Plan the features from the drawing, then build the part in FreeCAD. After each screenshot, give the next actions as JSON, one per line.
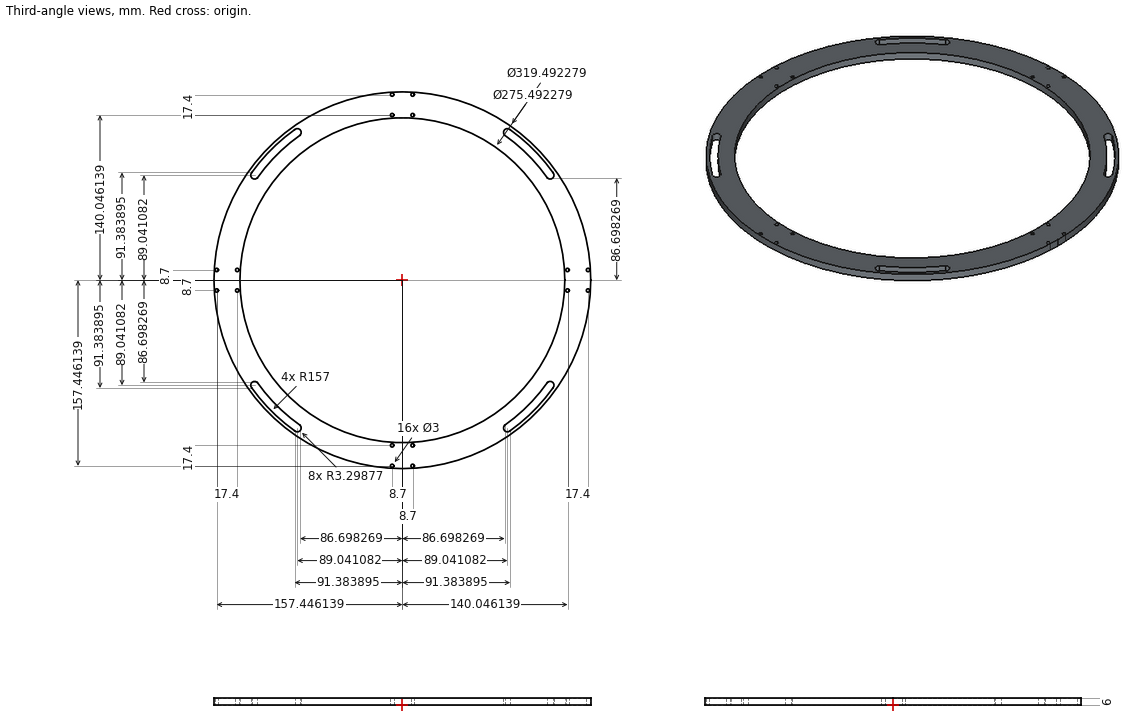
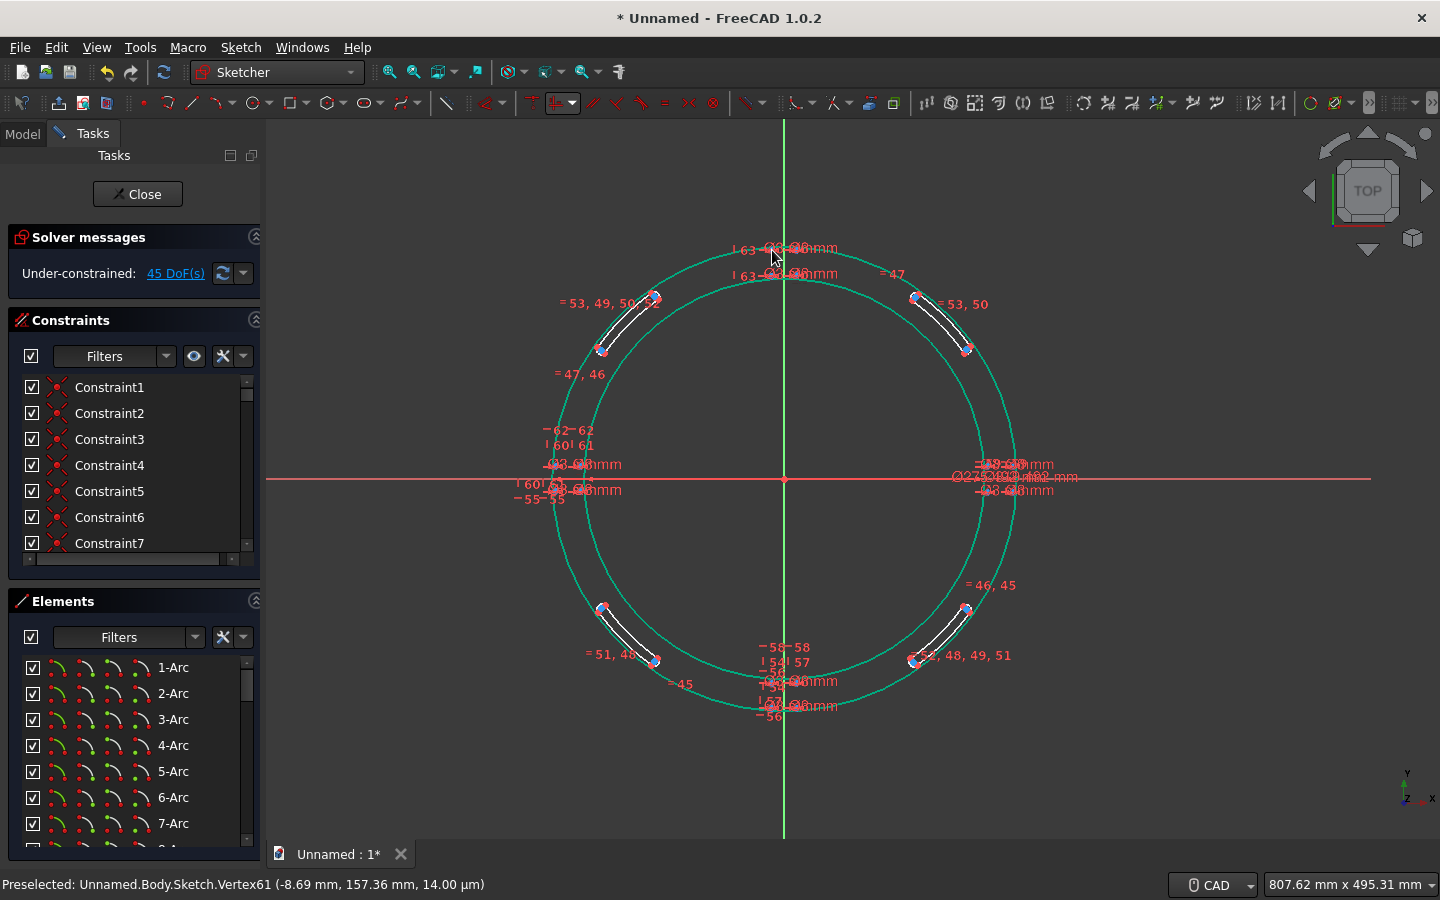
{"action": "left_click", "coordinate": [988, 492]}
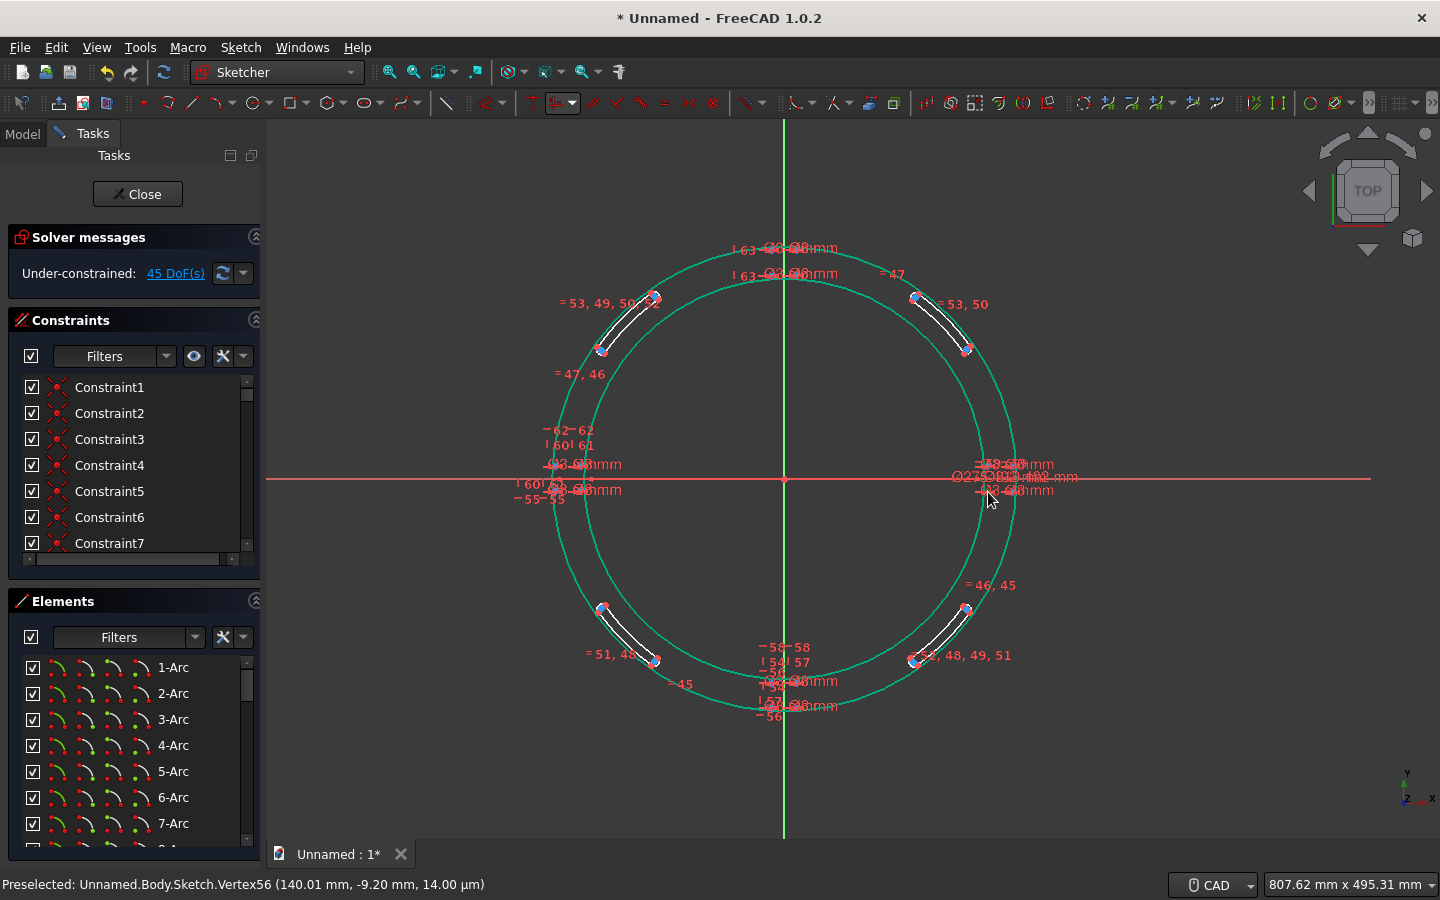
{"action": "left_click", "coordinate": [988, 467]}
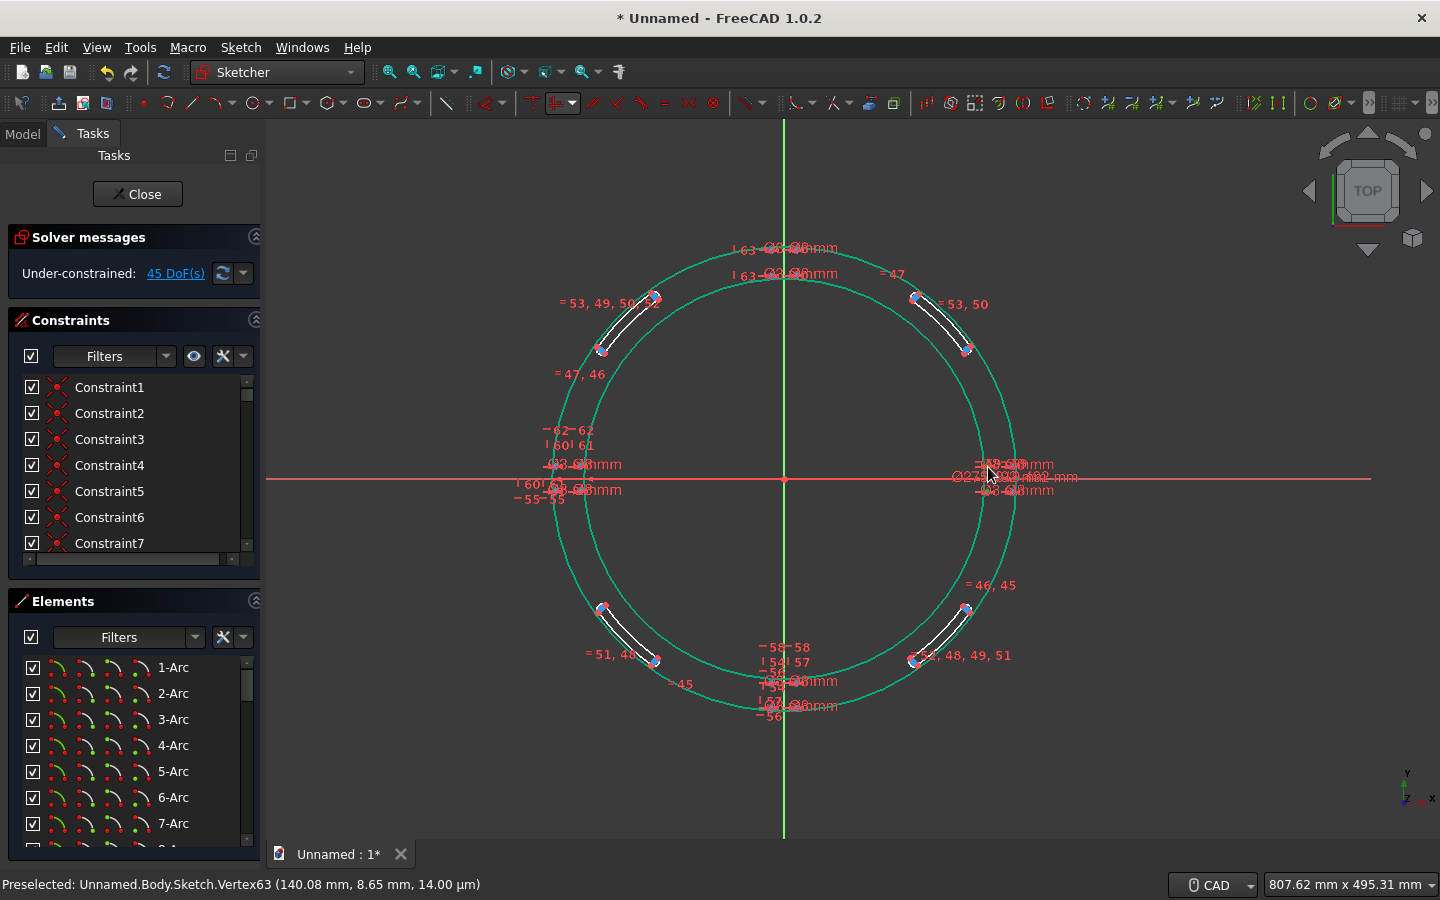
{"action": "key", "text": "v"}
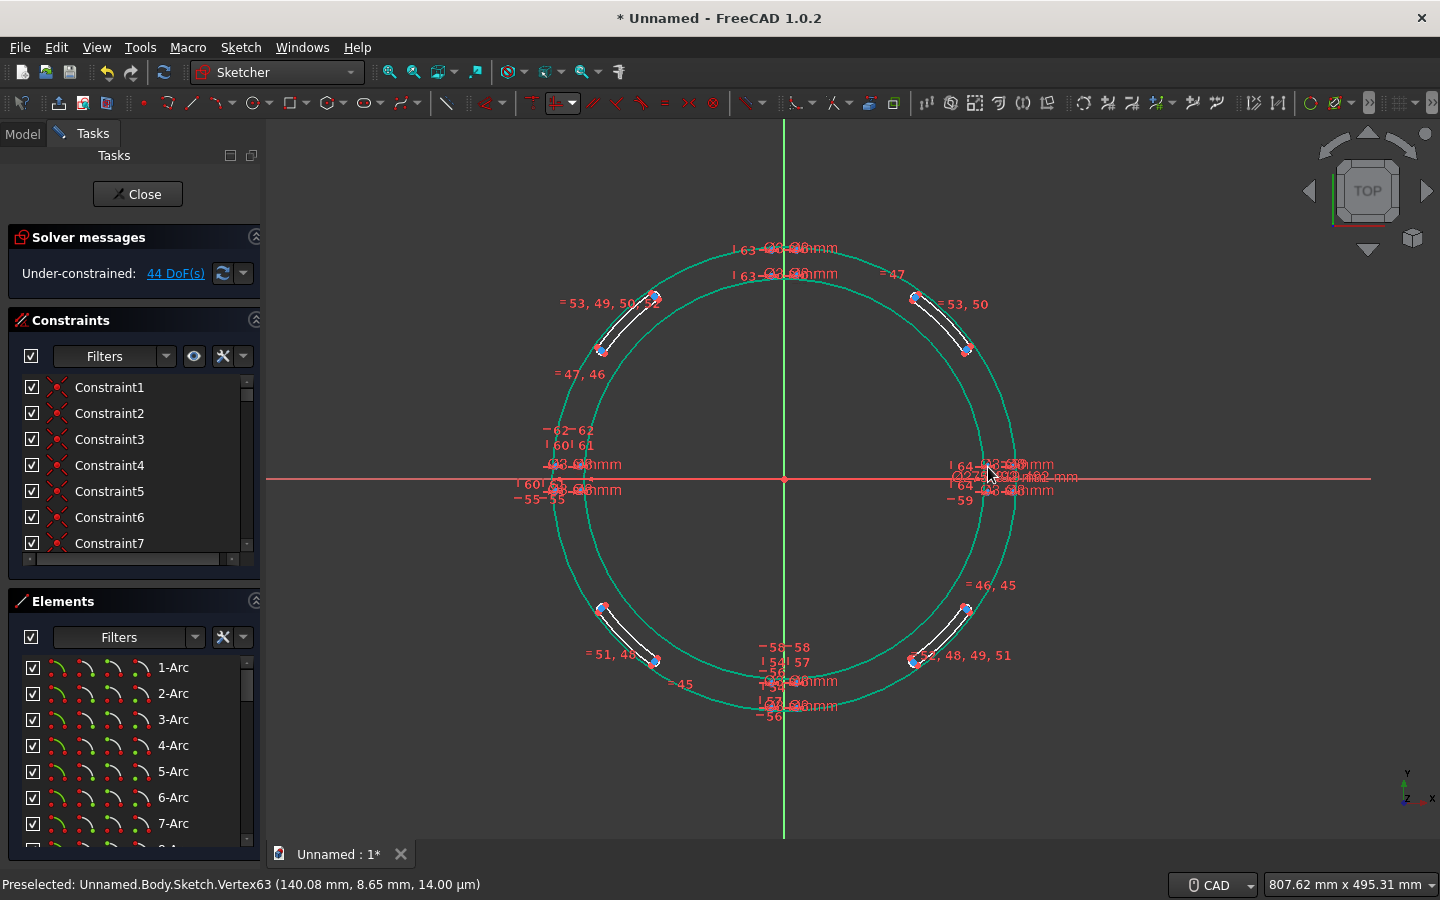
{"action": "left_click", "coordinate": [1013, 492]}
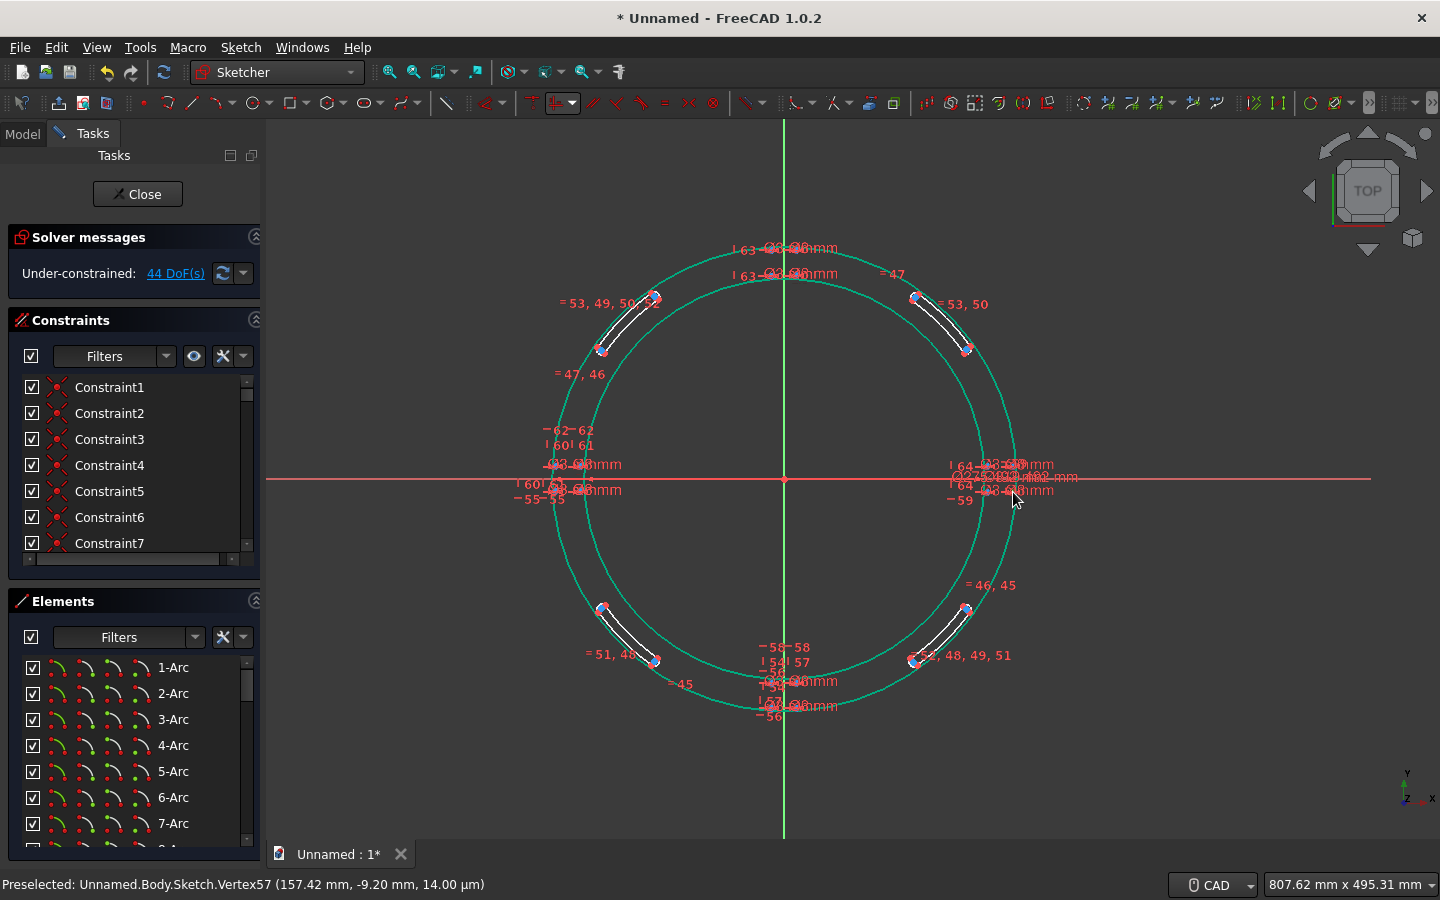
{"action": "scroll", "coordinate": [1013, 467], "scroll_direction": "up", "scroll_amount": 4}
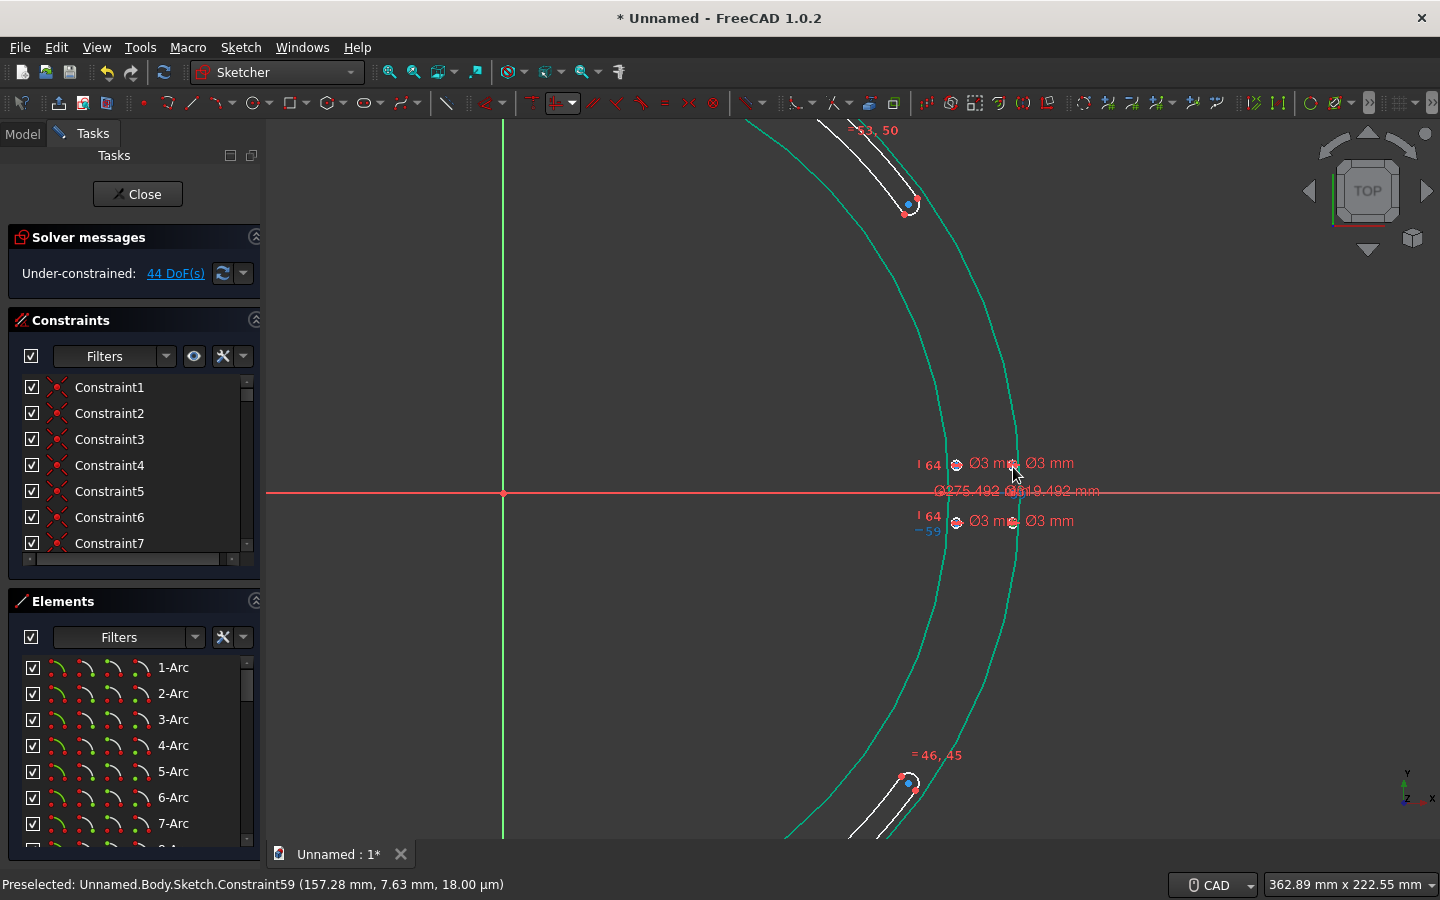
{"action": "left_click", "coordinate": [1013, 465]}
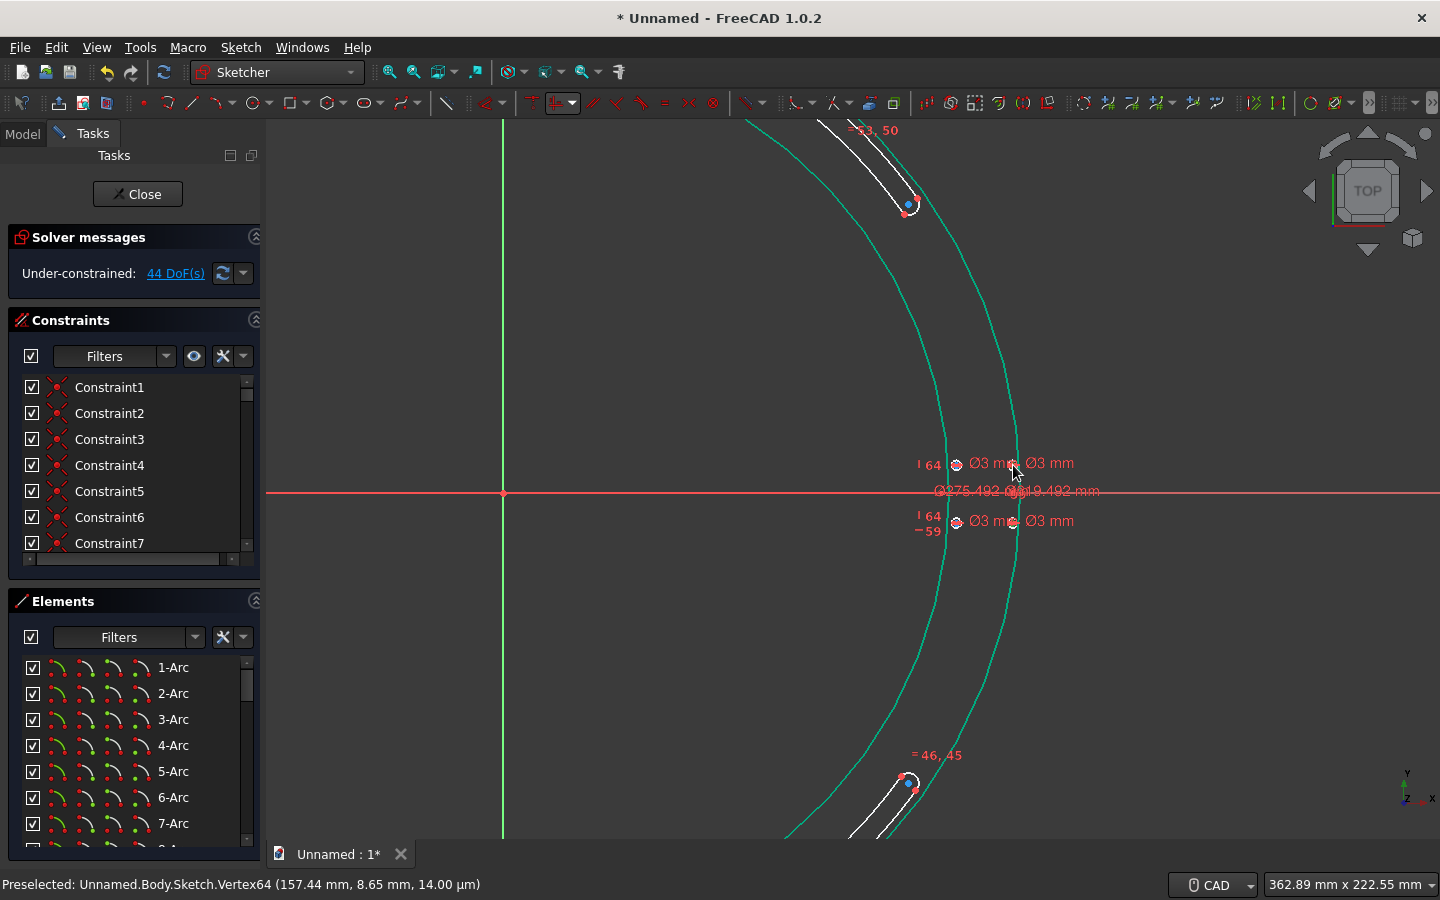
{"action": "key", "text": "v"}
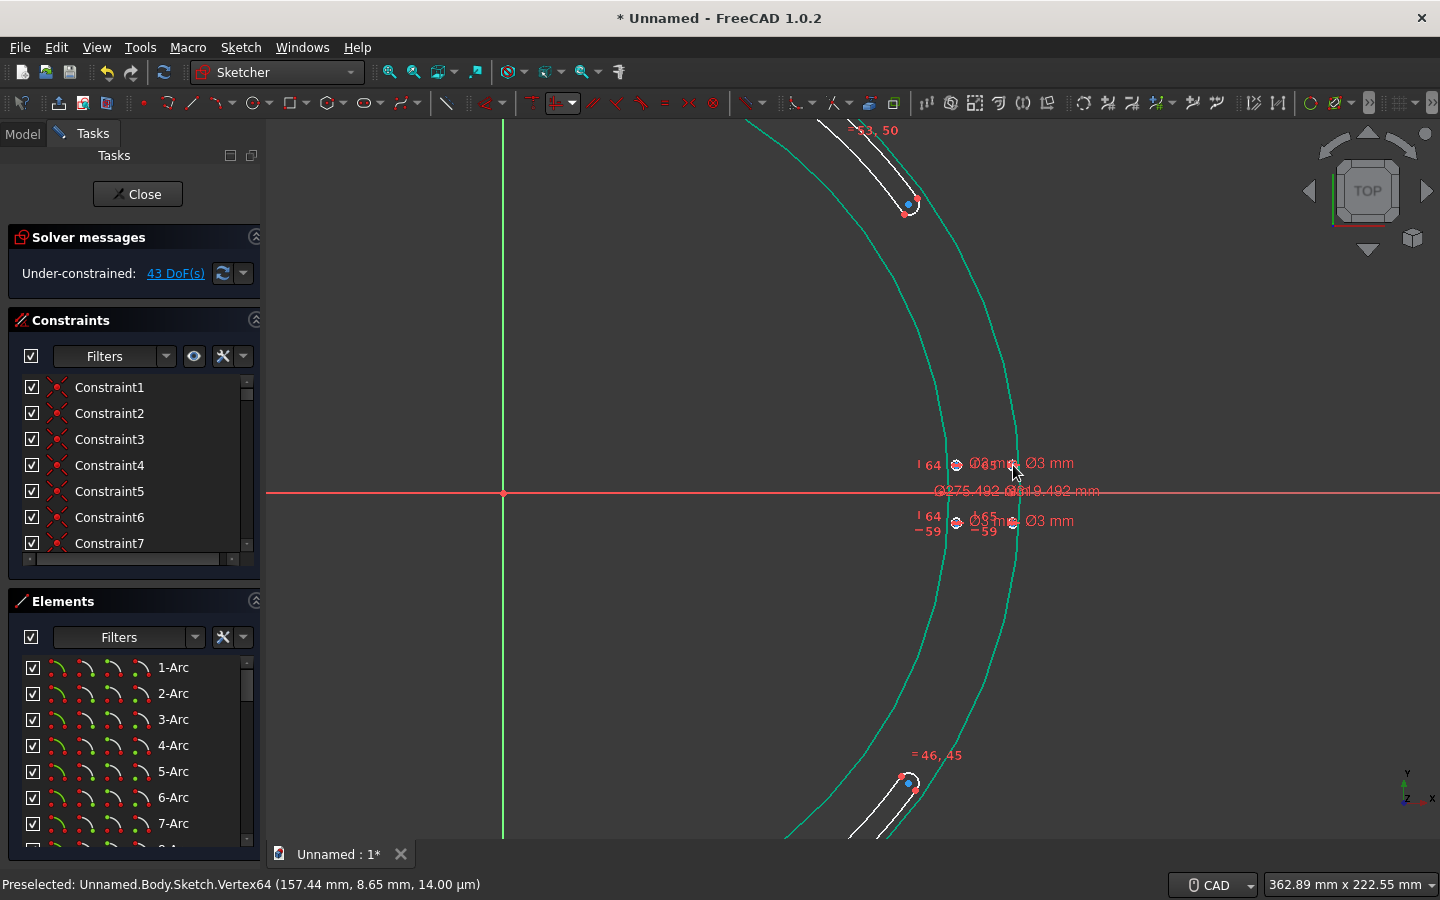
{"action": "left_click", "coordinate": [956, 465]}